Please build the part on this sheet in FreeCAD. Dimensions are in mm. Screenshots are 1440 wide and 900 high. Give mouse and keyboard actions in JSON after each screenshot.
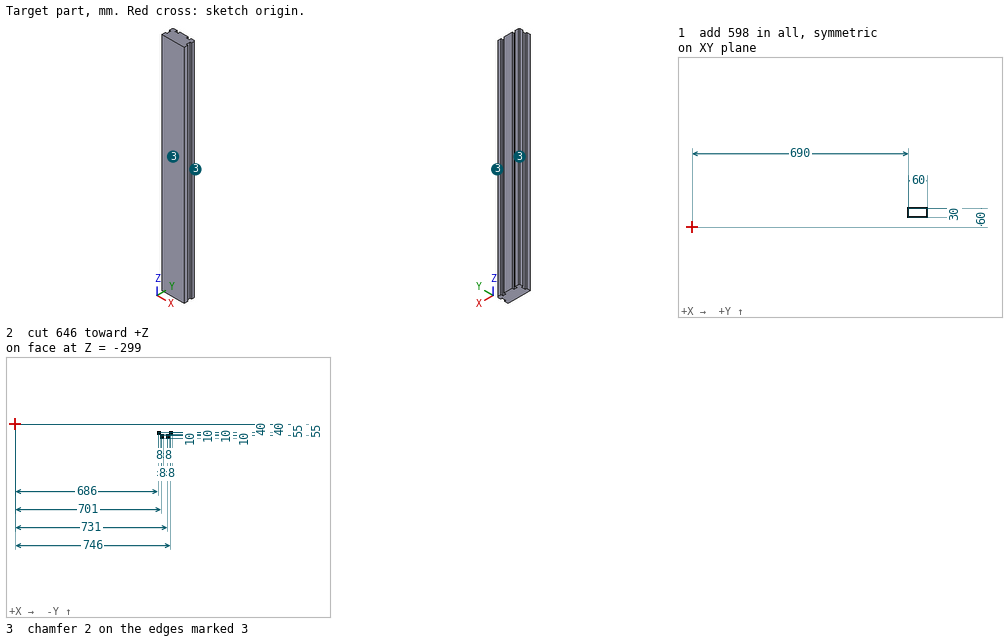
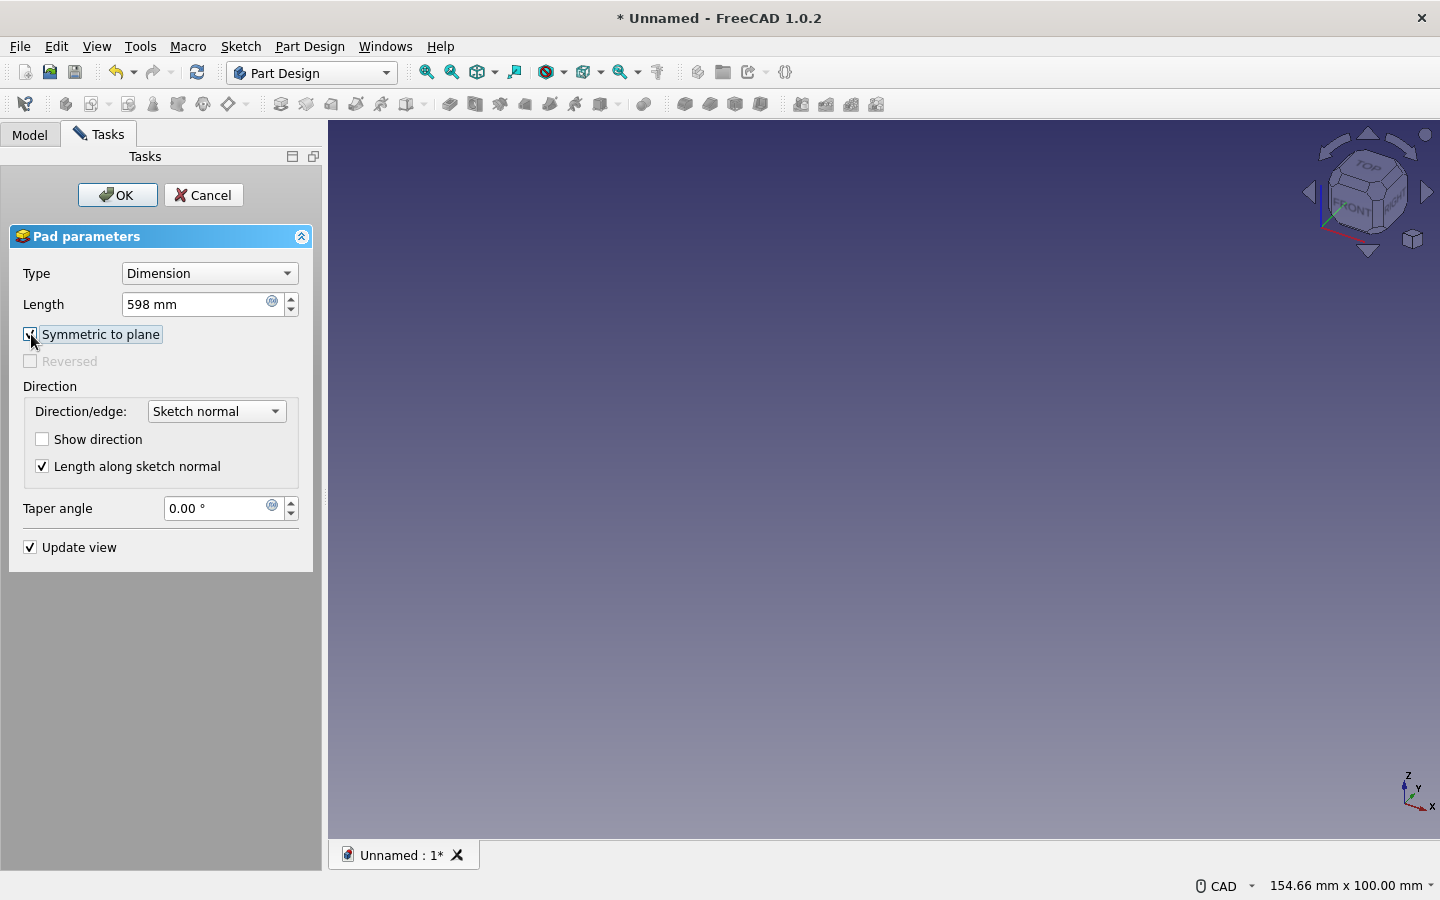
{"action": "left_click", "coordinate": [118, 195]}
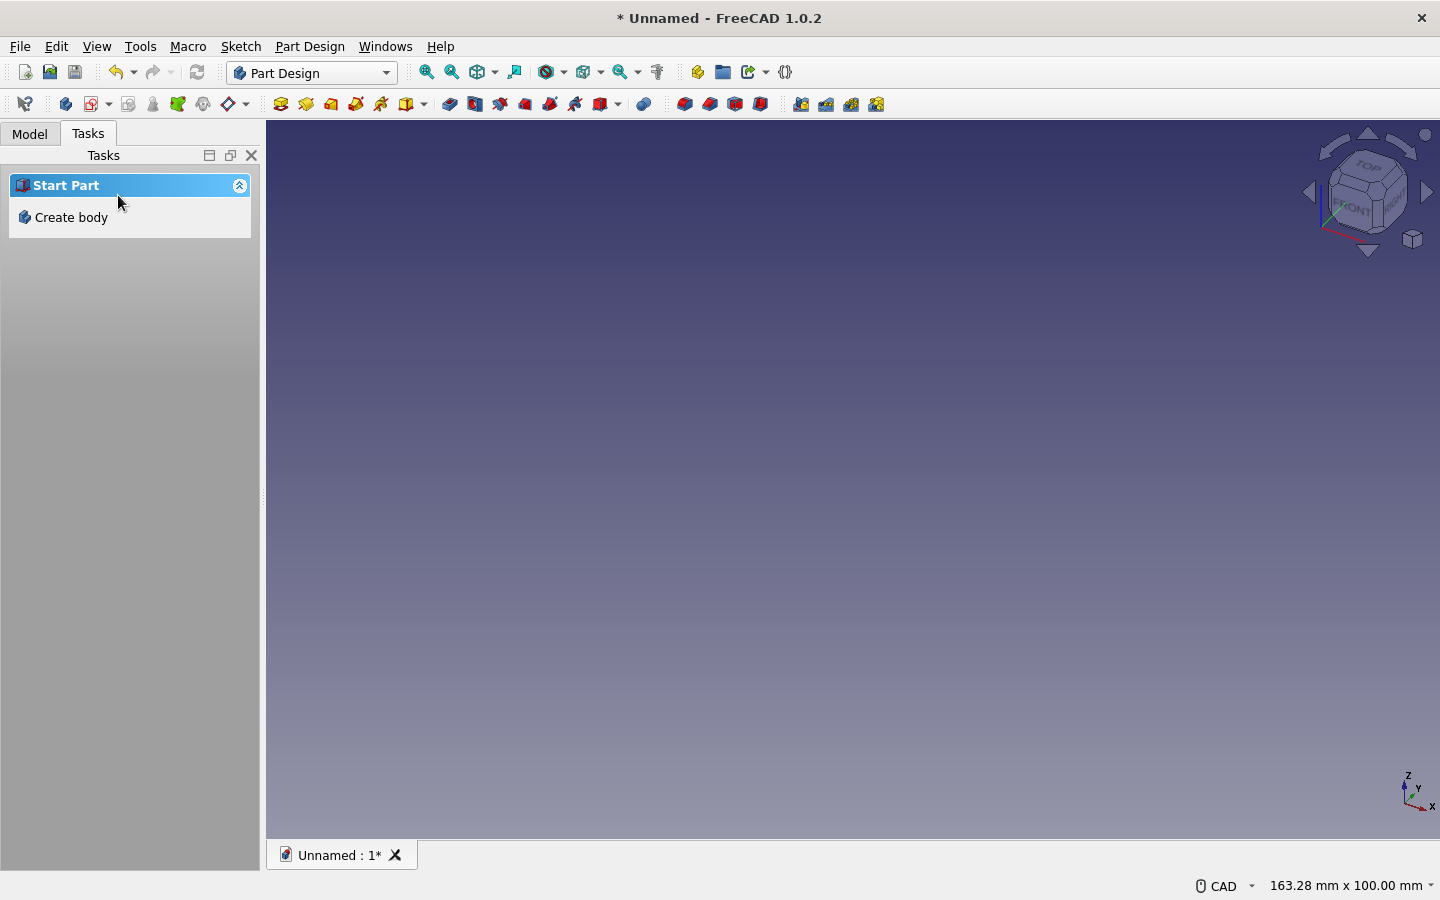
{"action": "left_click", "coordinate": [427, 72]}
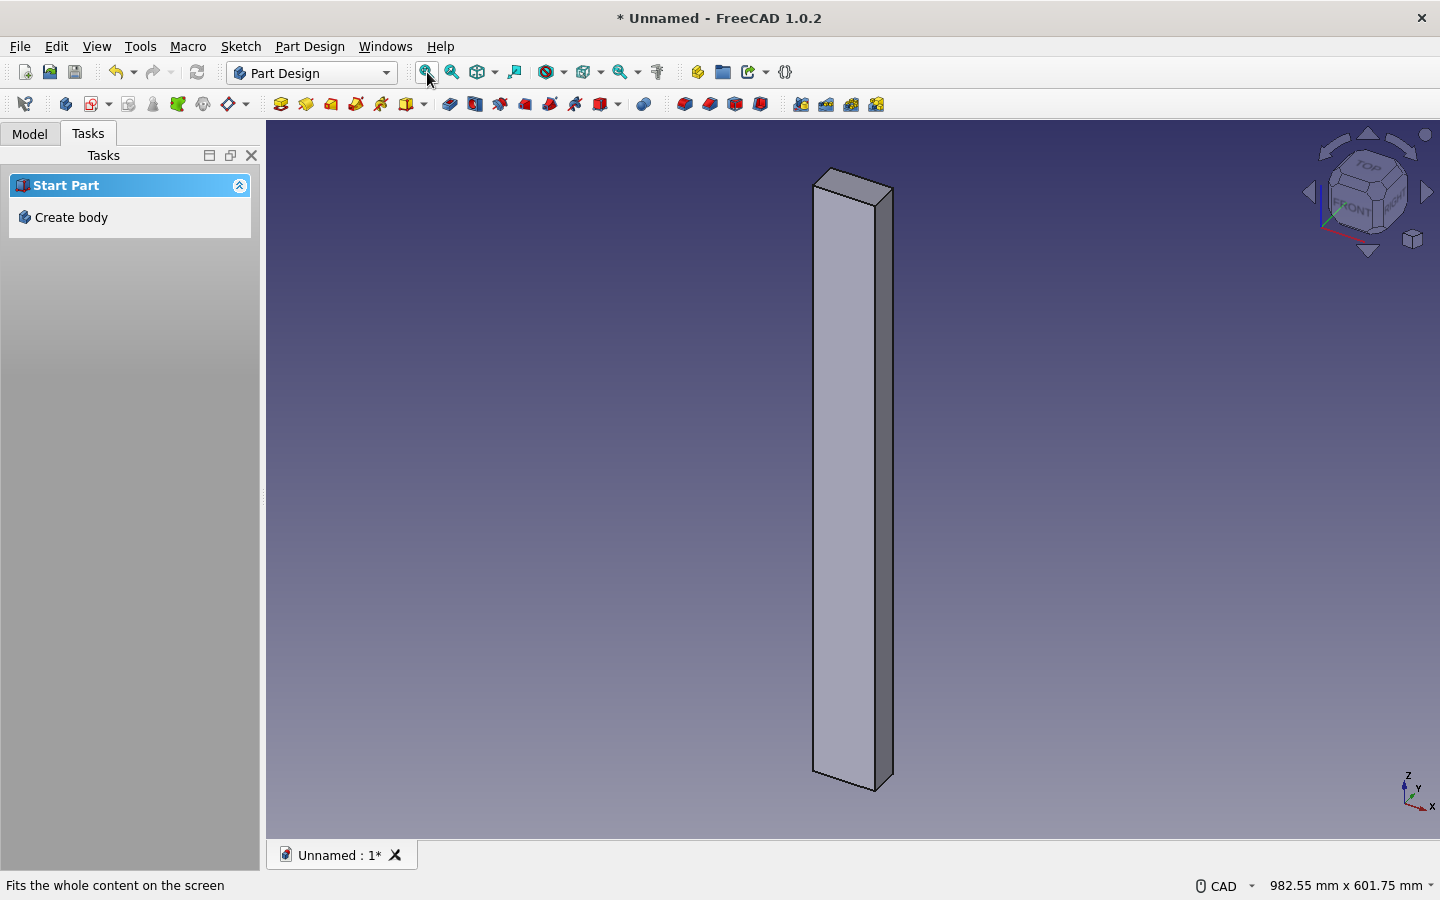
{"action": "key", "text": "5"}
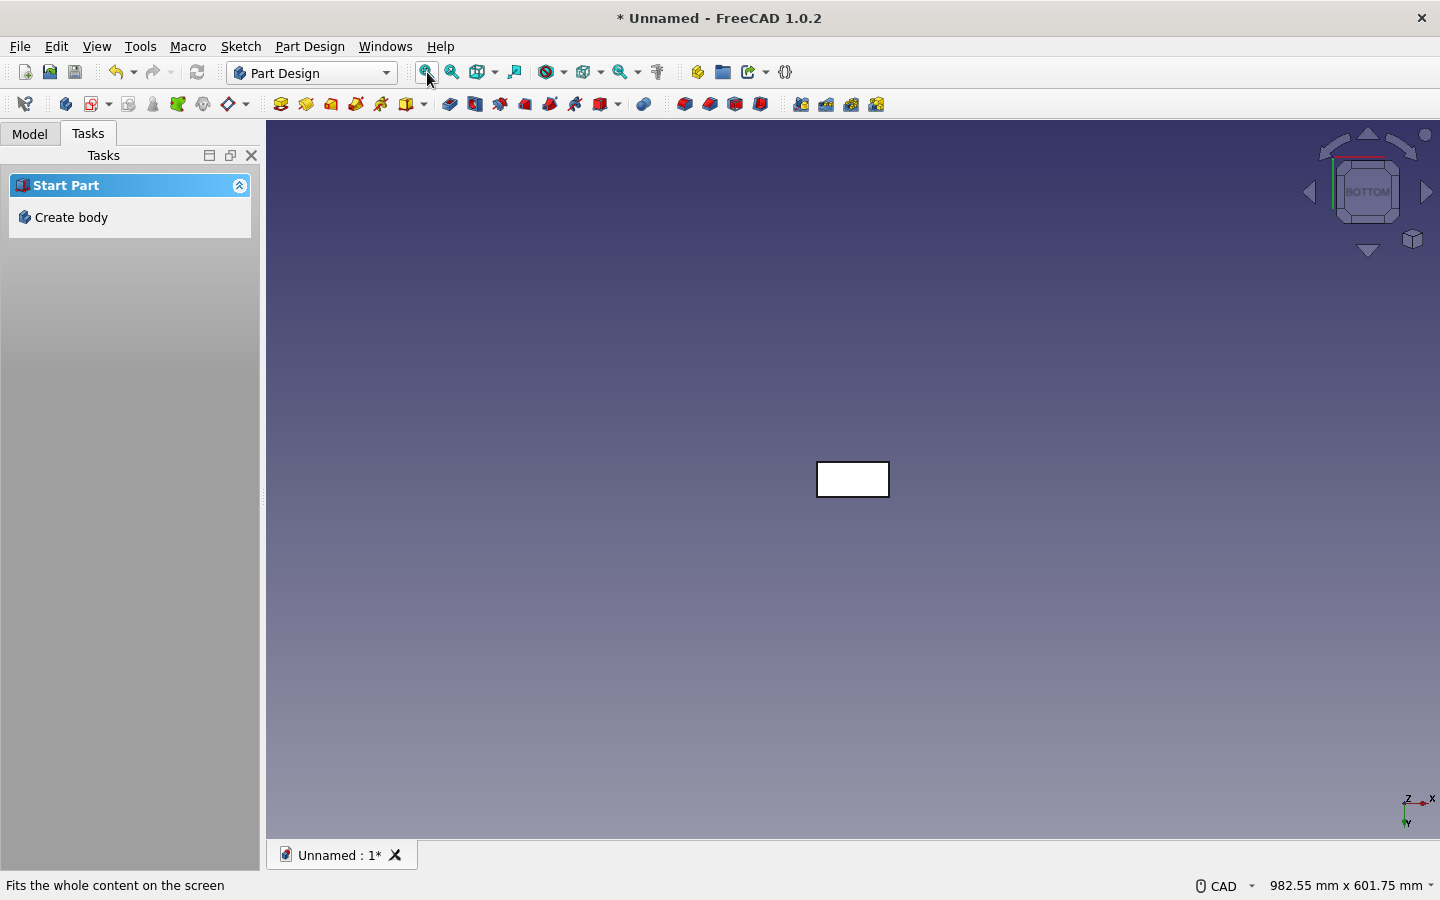
{"action": "left_click", "coordinate": [427, 72]}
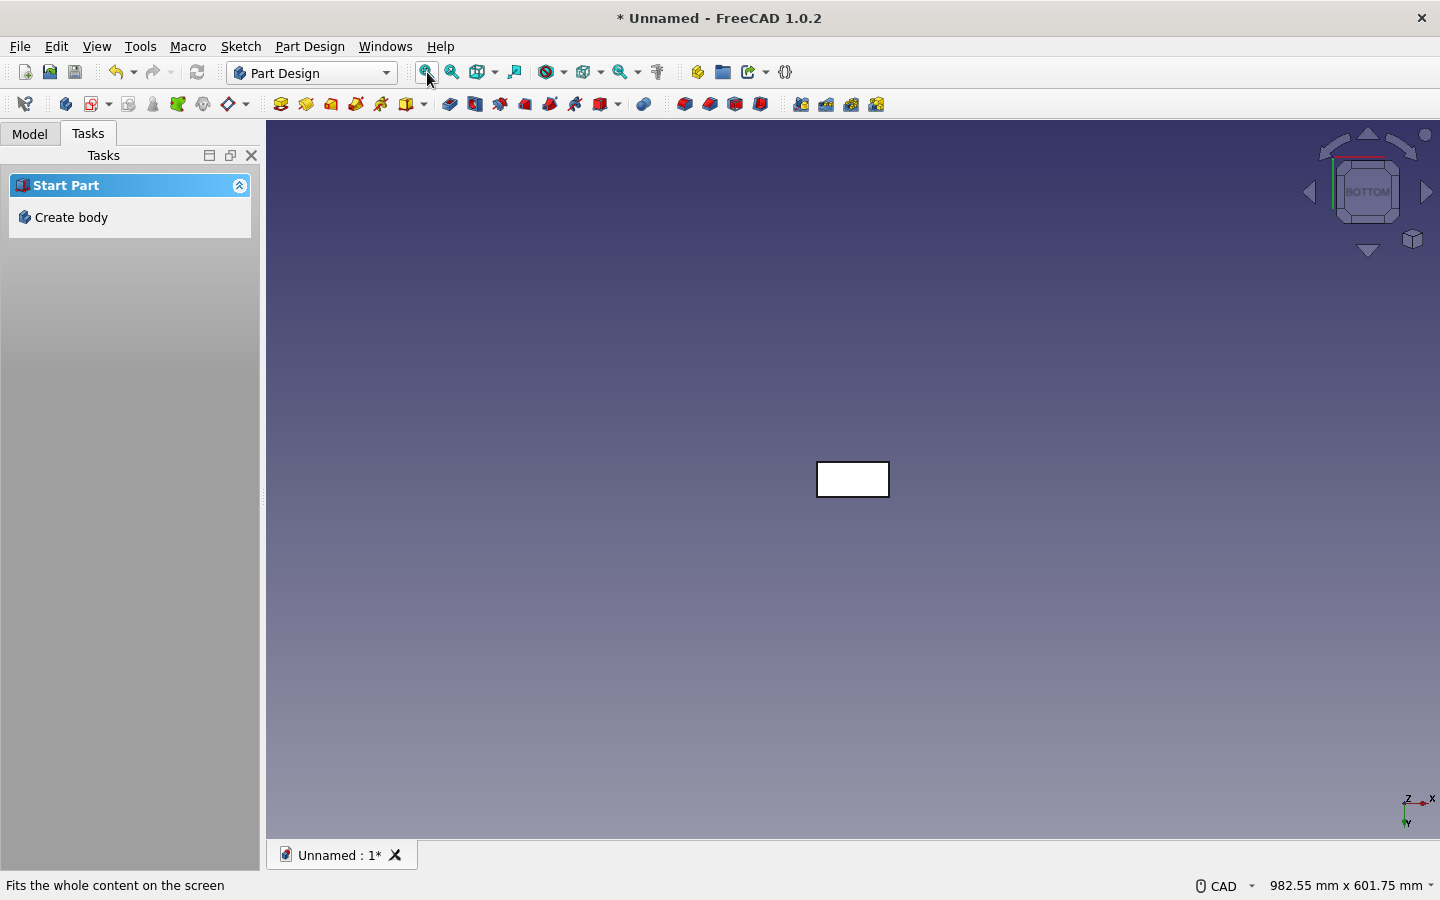
{"action": "left_click", "coordinate": [863, 478]}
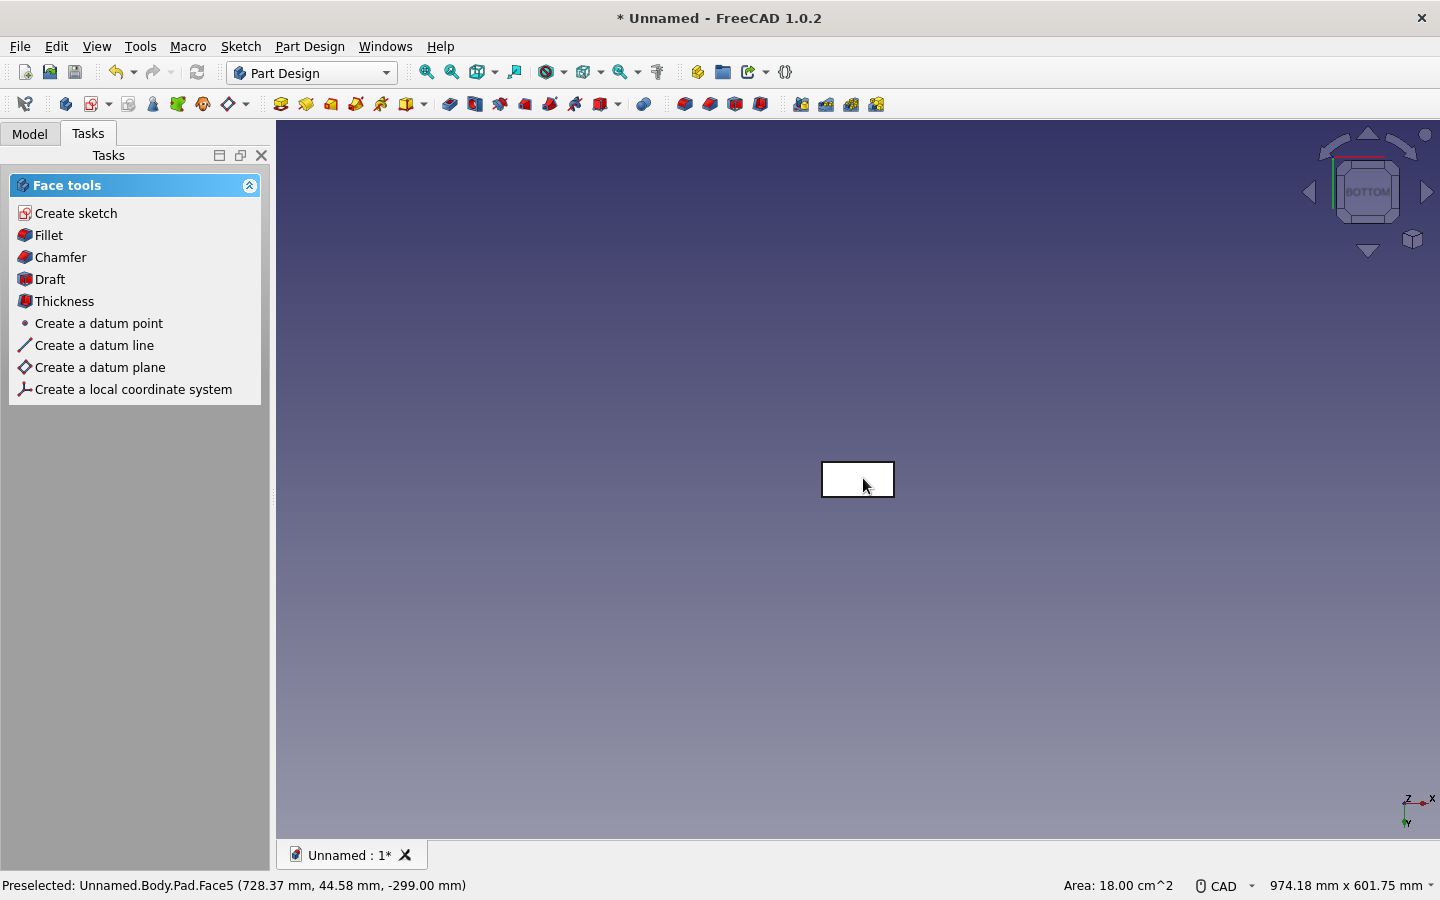
{"action": "left_click", "coordinate": [90, 104]}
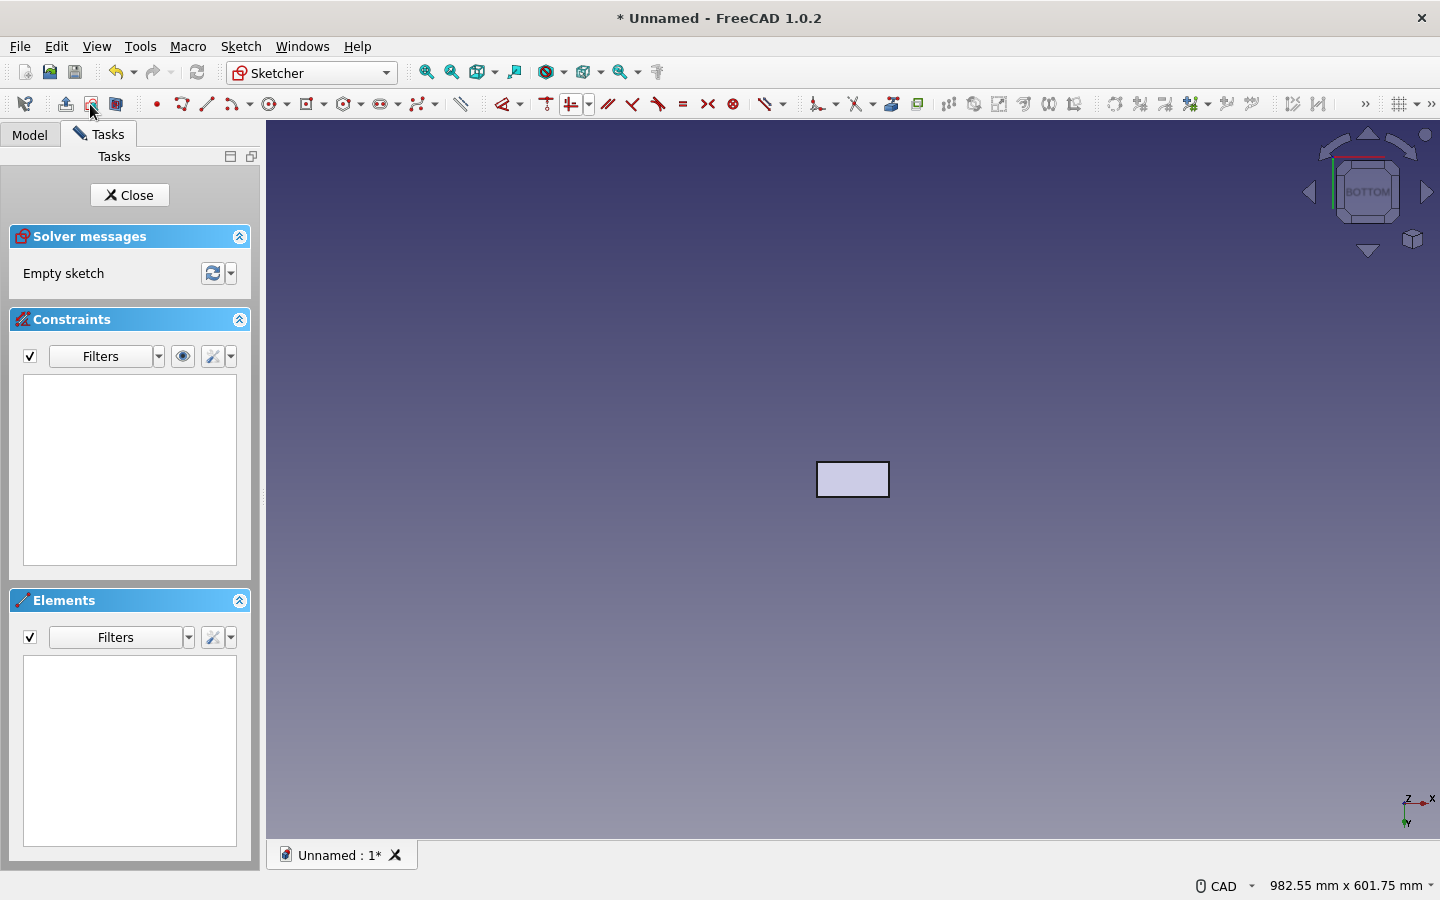
{"action": "scroll", "coordinate": [862, 490], "scroll_direction": "up", "scroll_amount": 11}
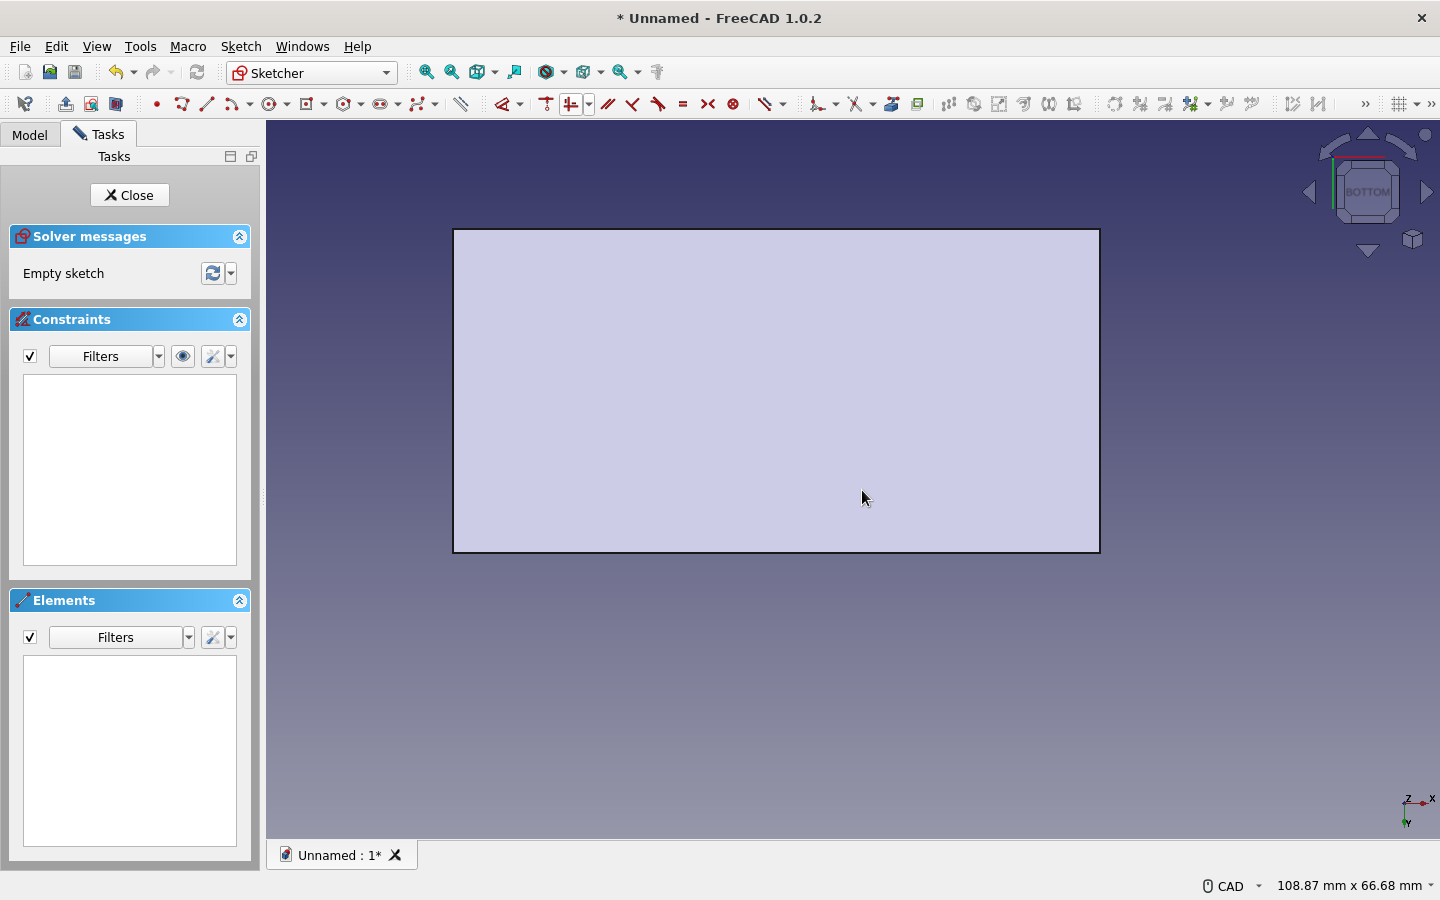
{"action": "left_click", "coordinate": [324, 104]}